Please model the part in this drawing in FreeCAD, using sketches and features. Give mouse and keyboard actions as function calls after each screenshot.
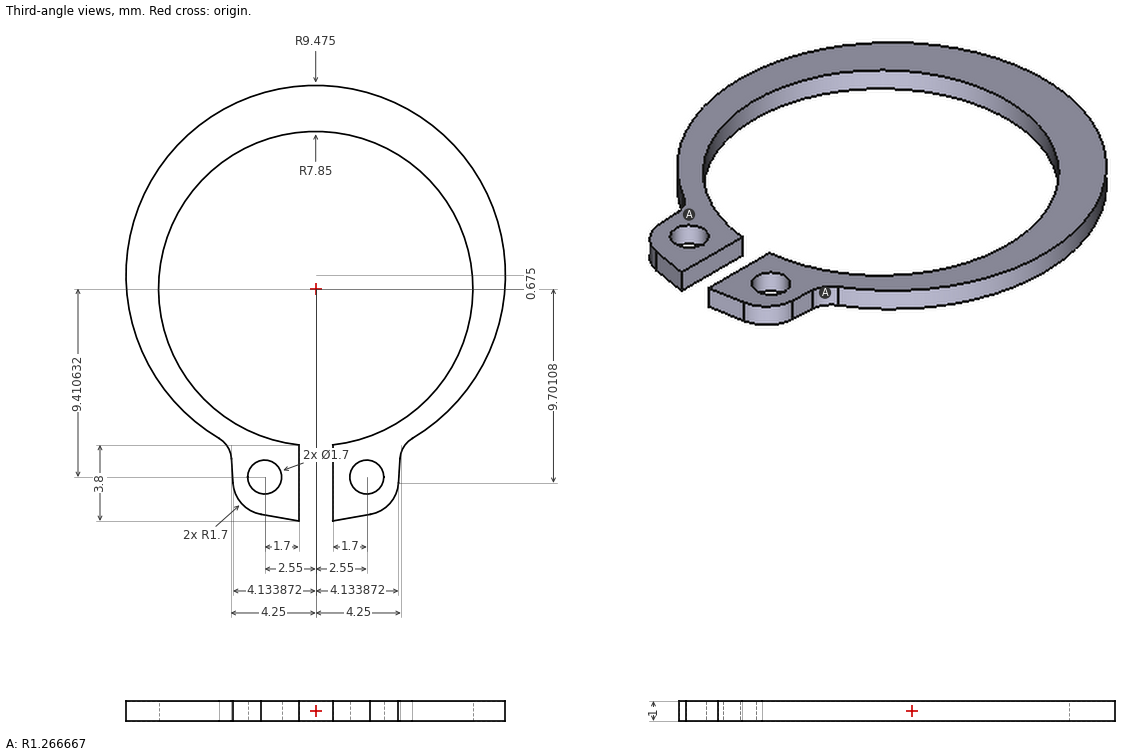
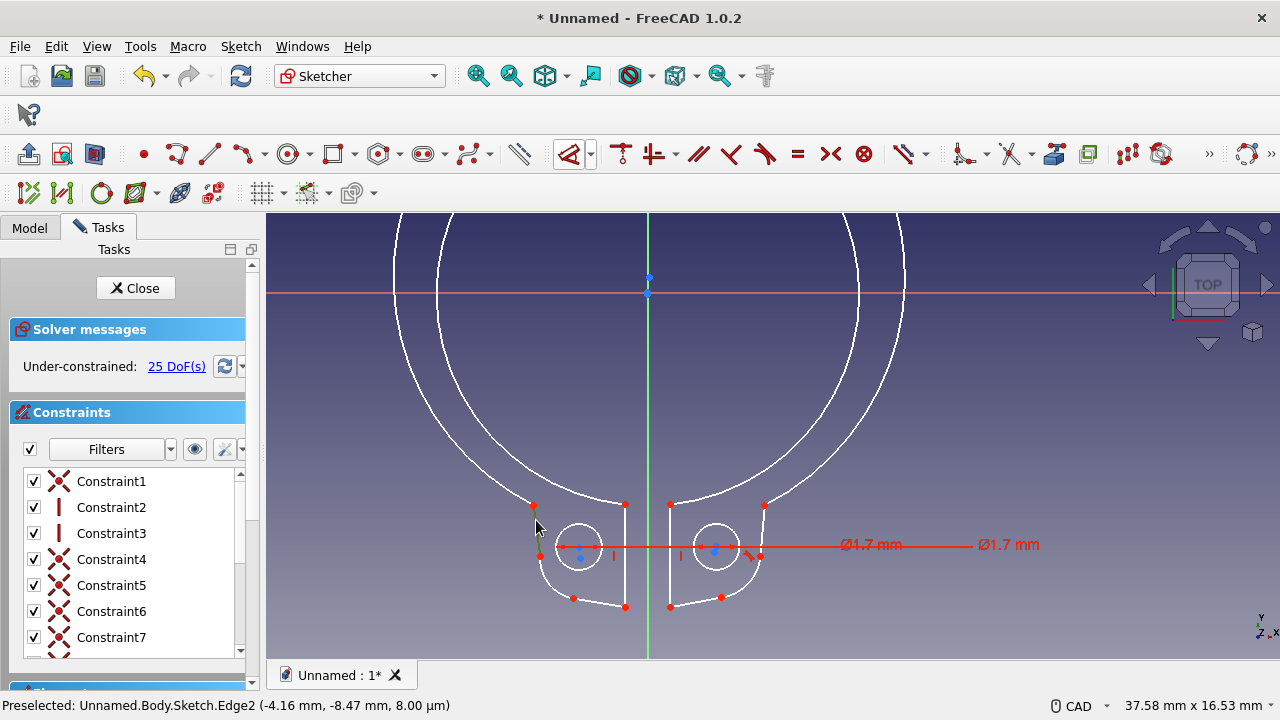
click(543, 574)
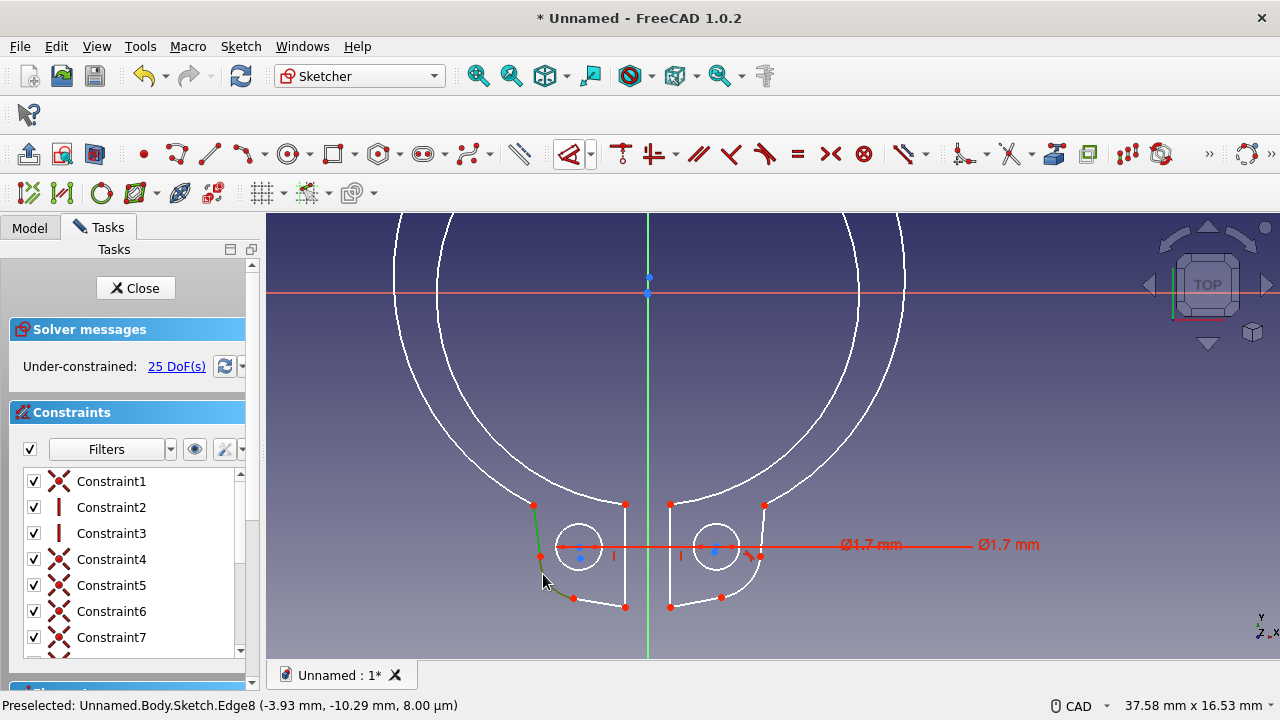
click(765, 154)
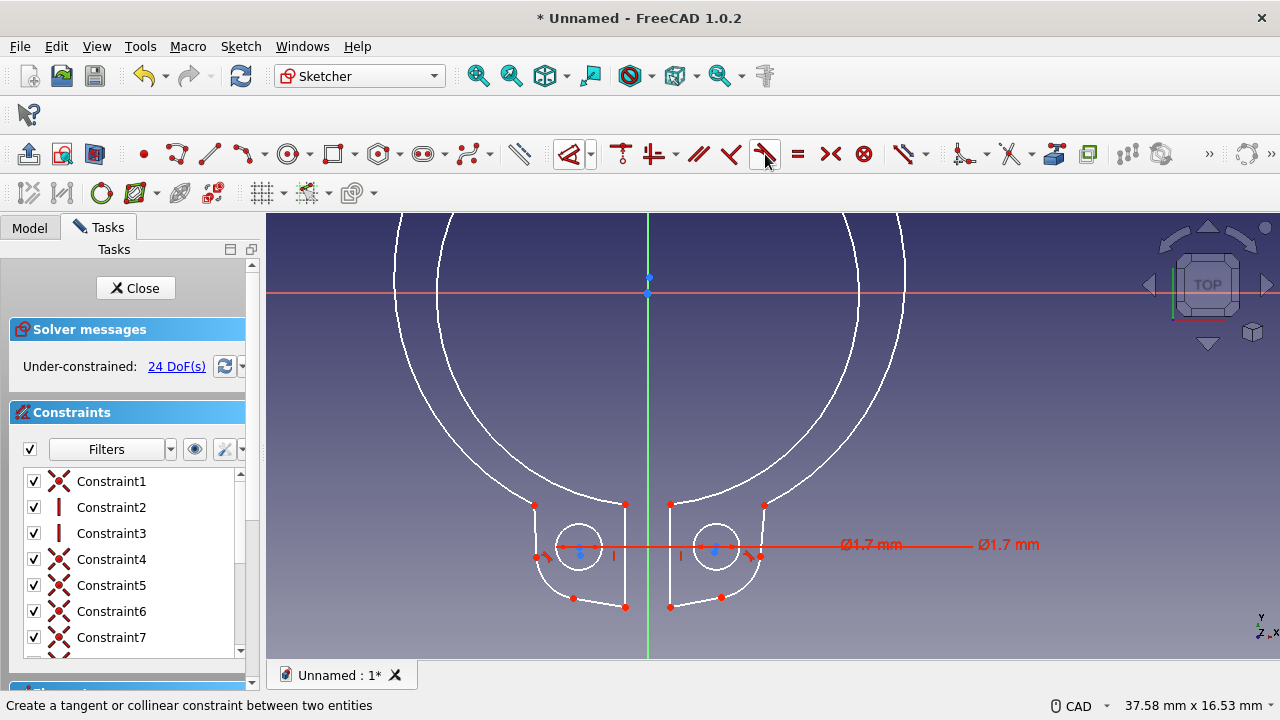
click(589, 601)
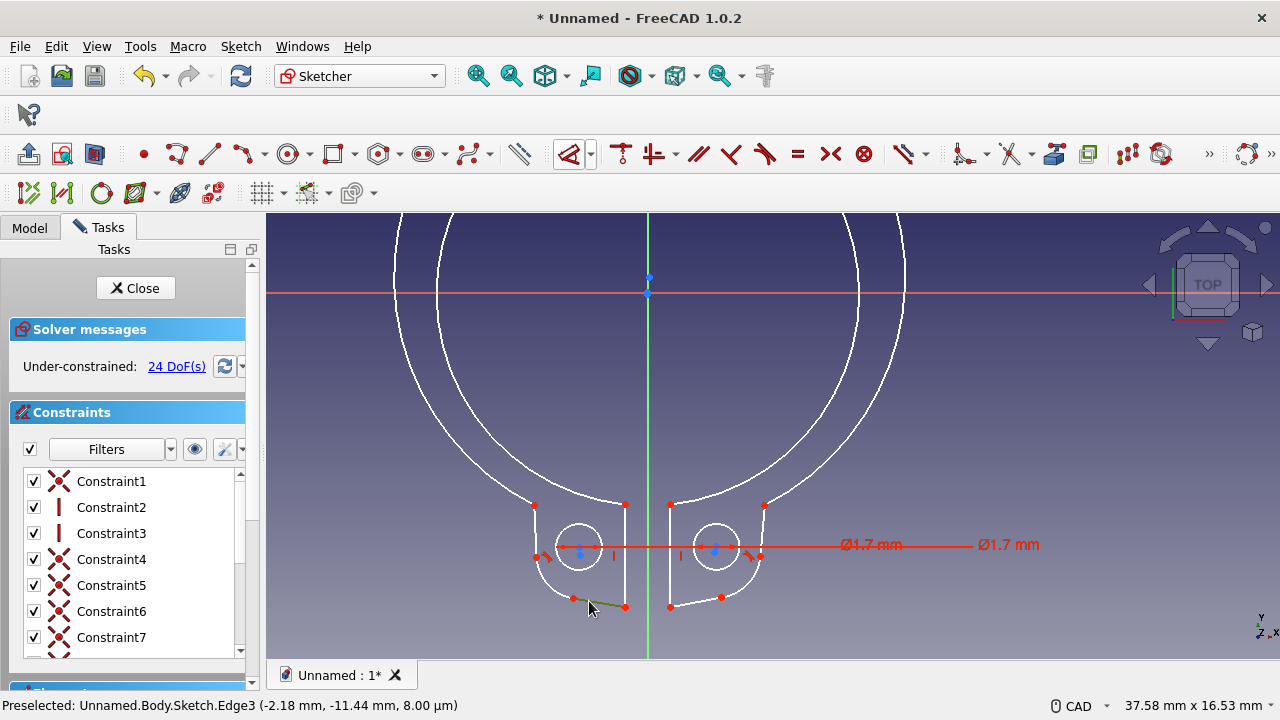
click(541, 575)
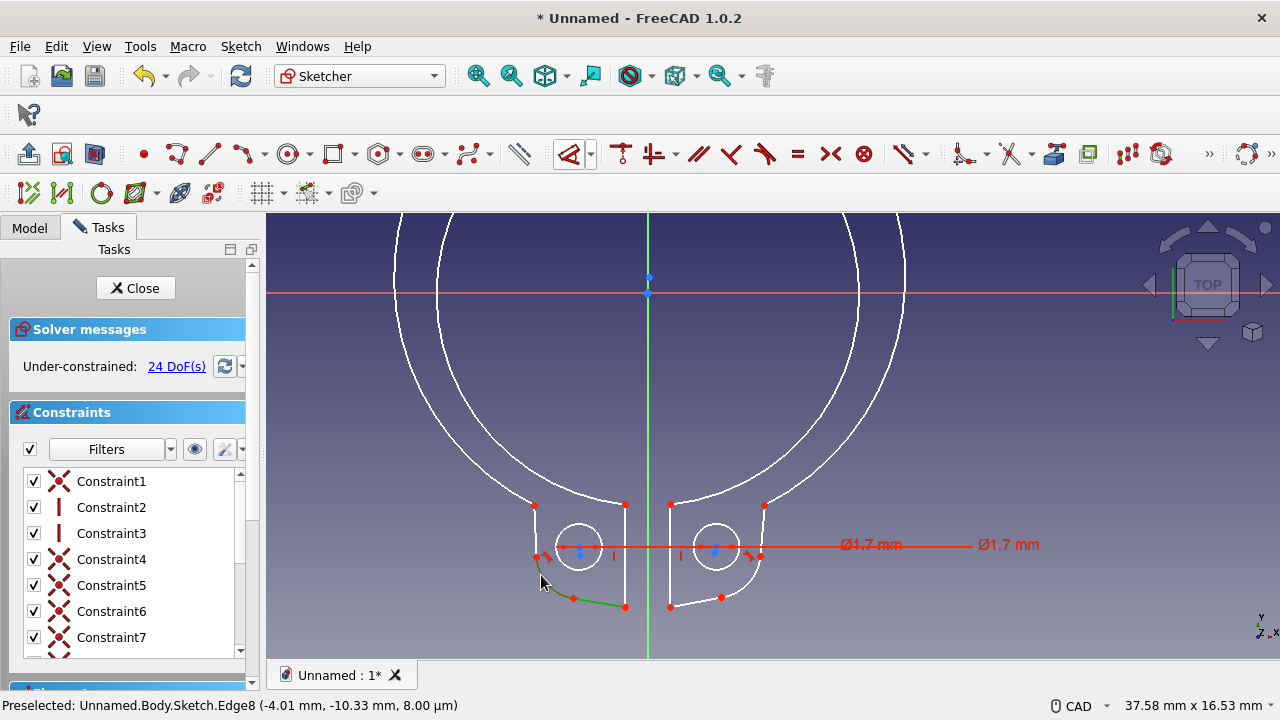
click(765, 154)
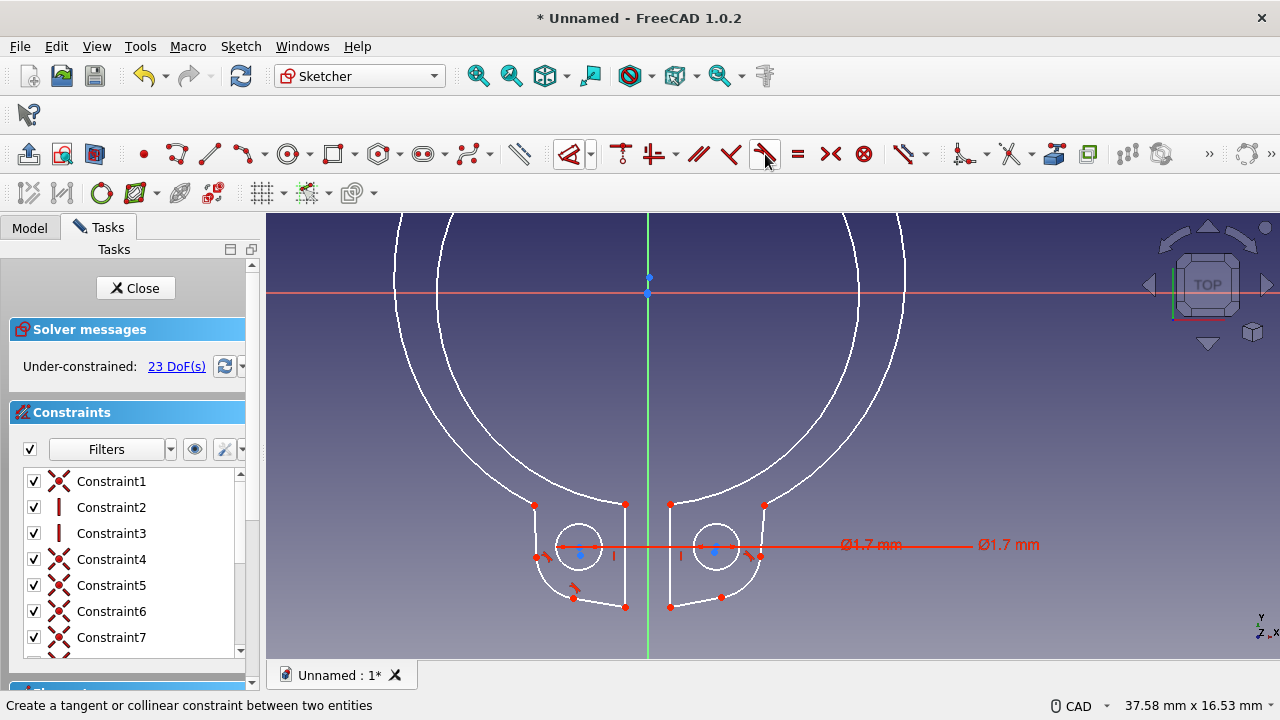
click(686, 604)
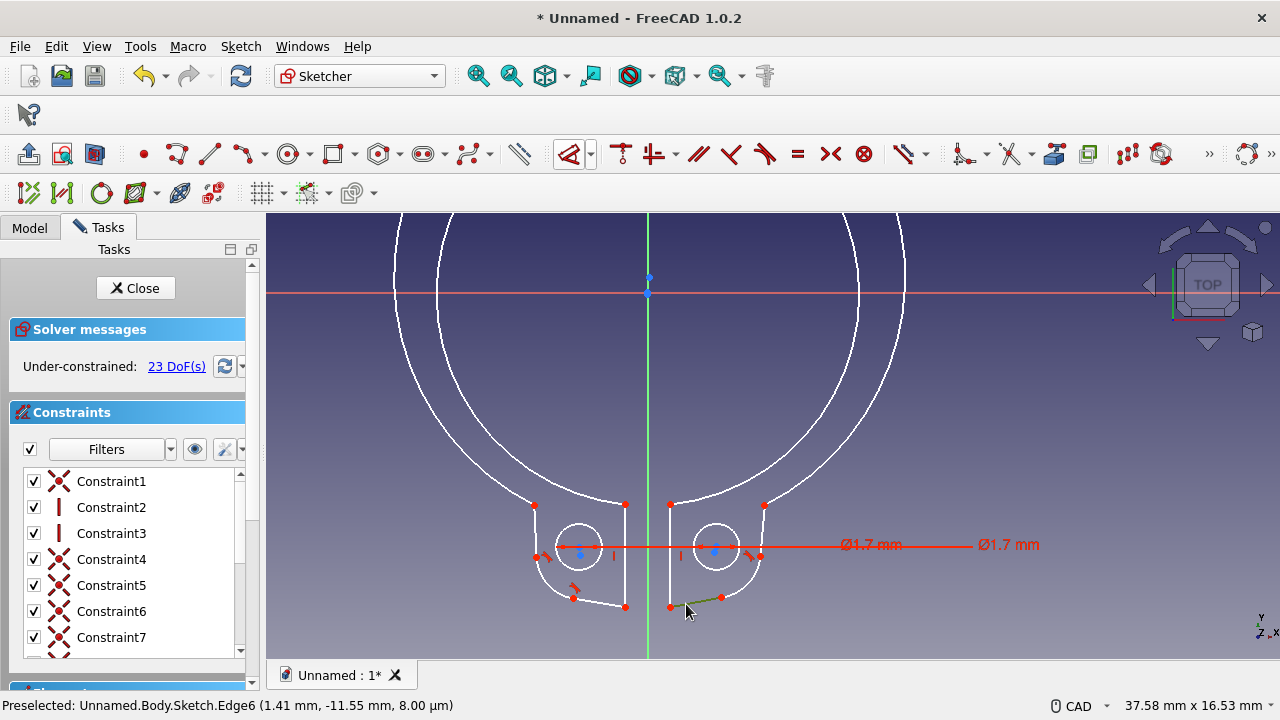
click(739, 591)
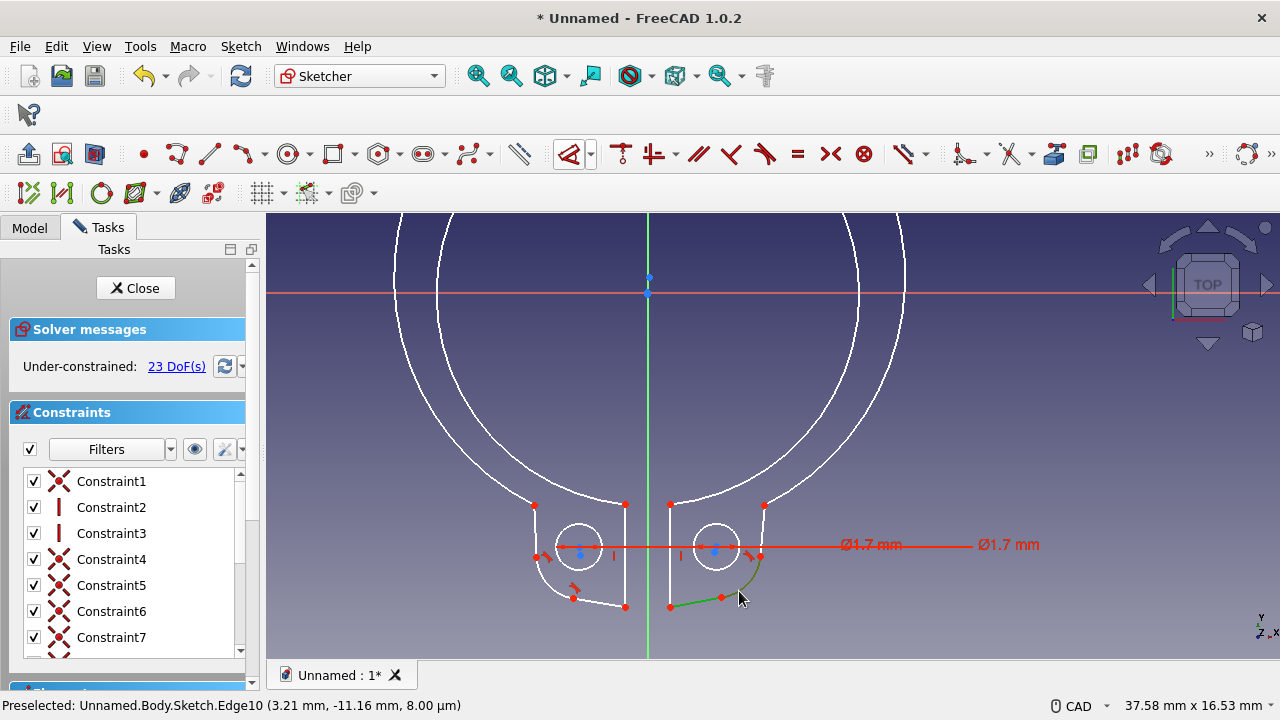
click(765, 154)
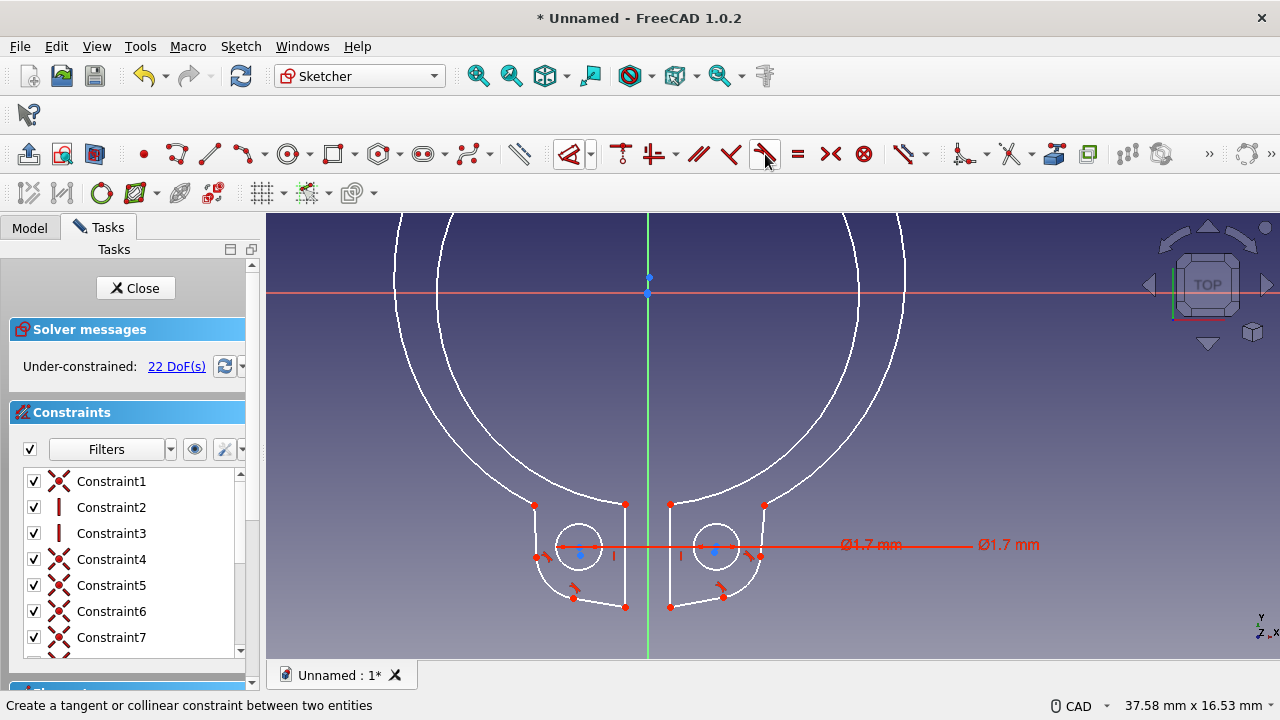
scroll(648, 294, up, 3)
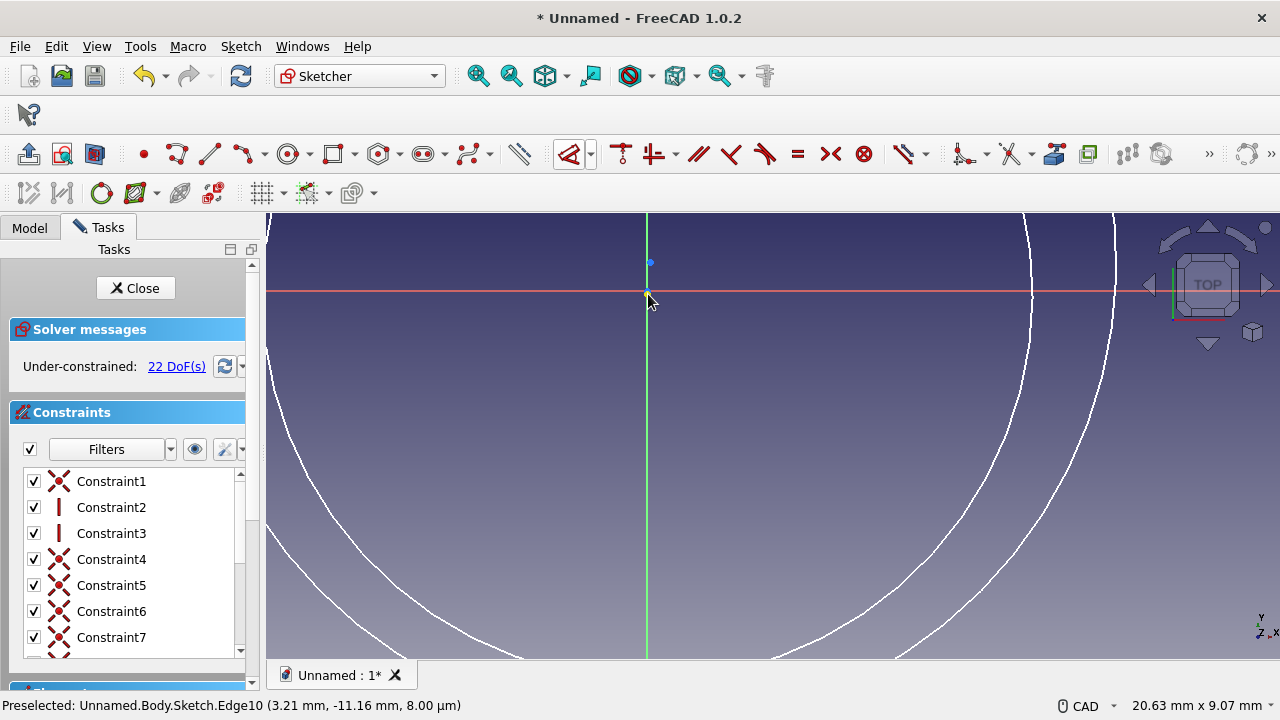
drag(637, 281, 657, 305)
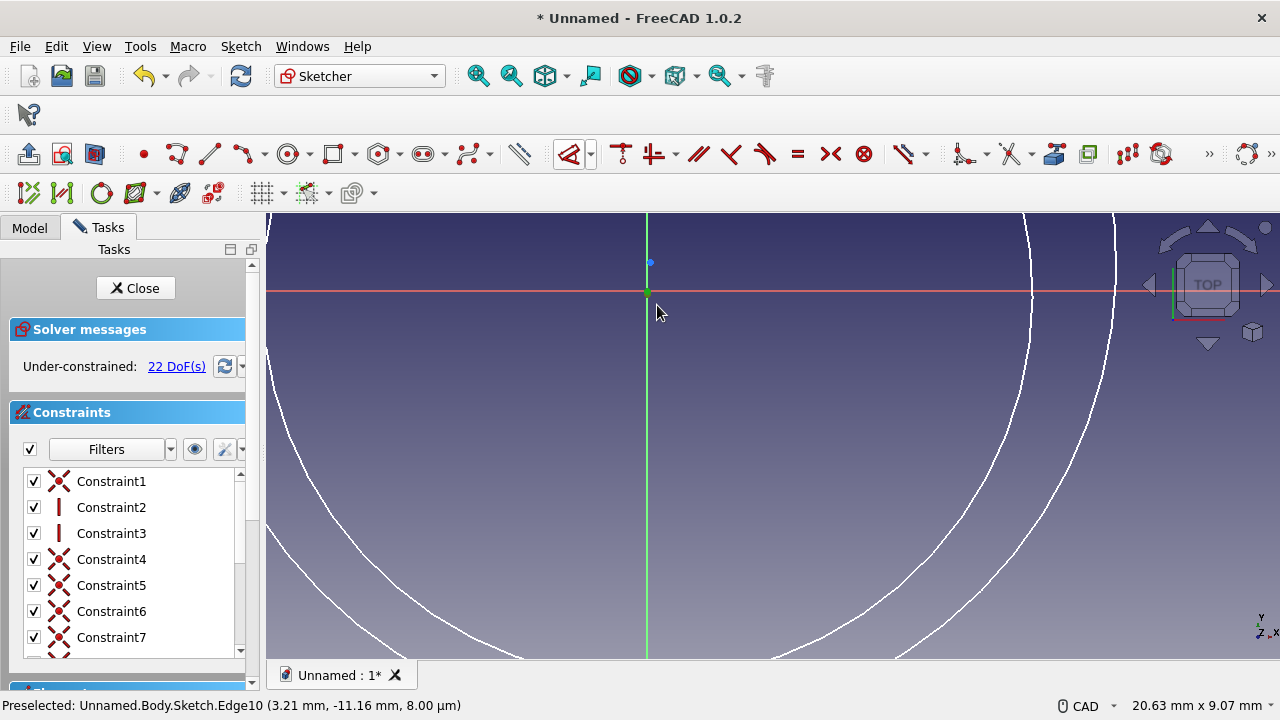
click(621, 154)